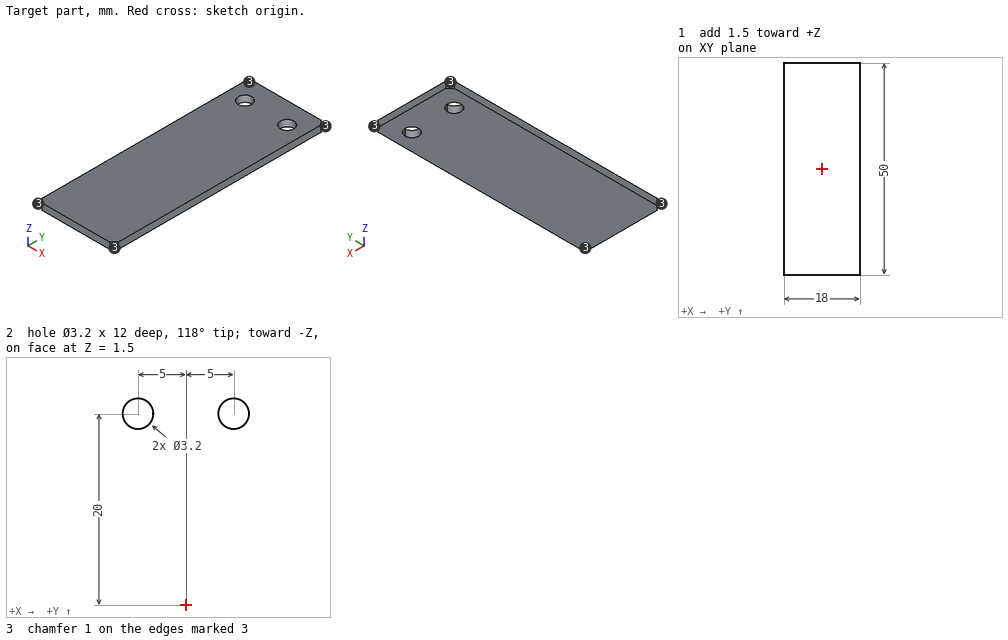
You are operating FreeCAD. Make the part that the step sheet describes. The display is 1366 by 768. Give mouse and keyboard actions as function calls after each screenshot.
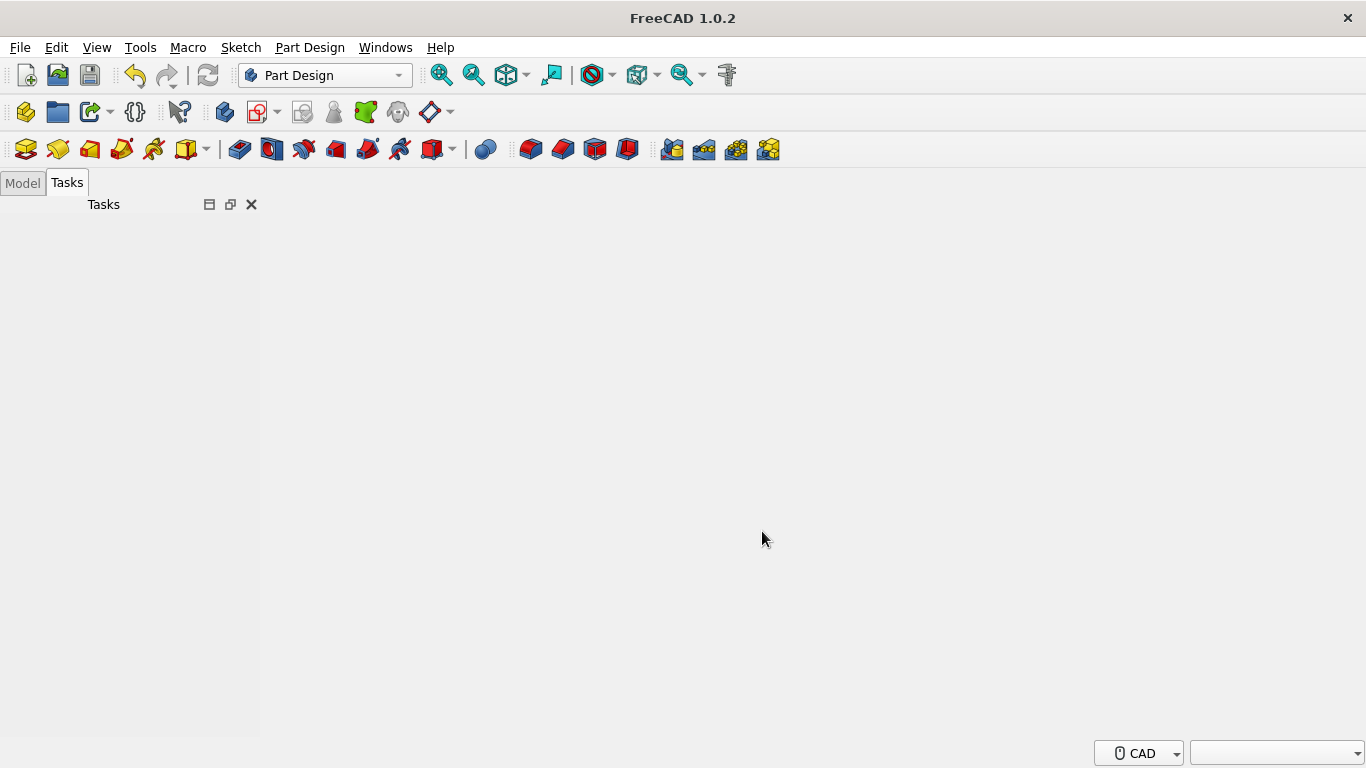
click(26, 76)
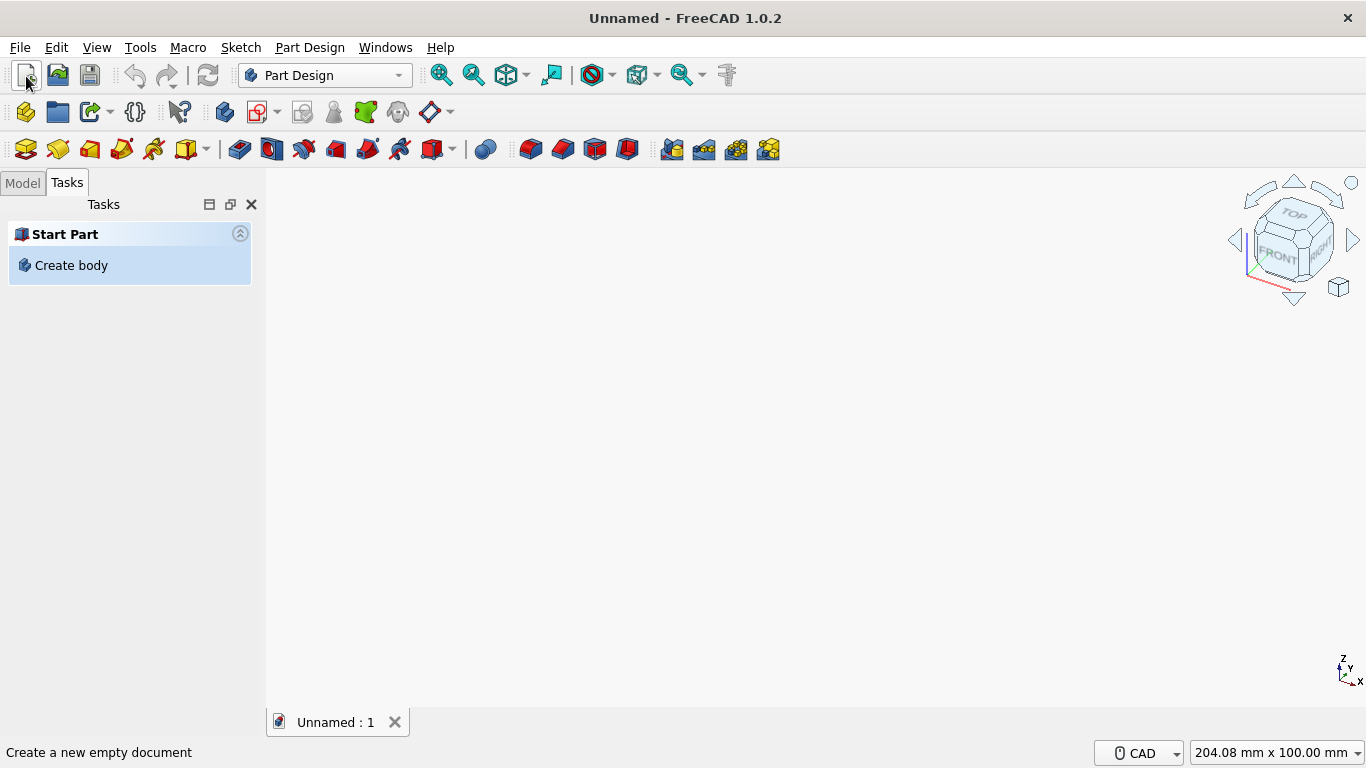
click(258, 112)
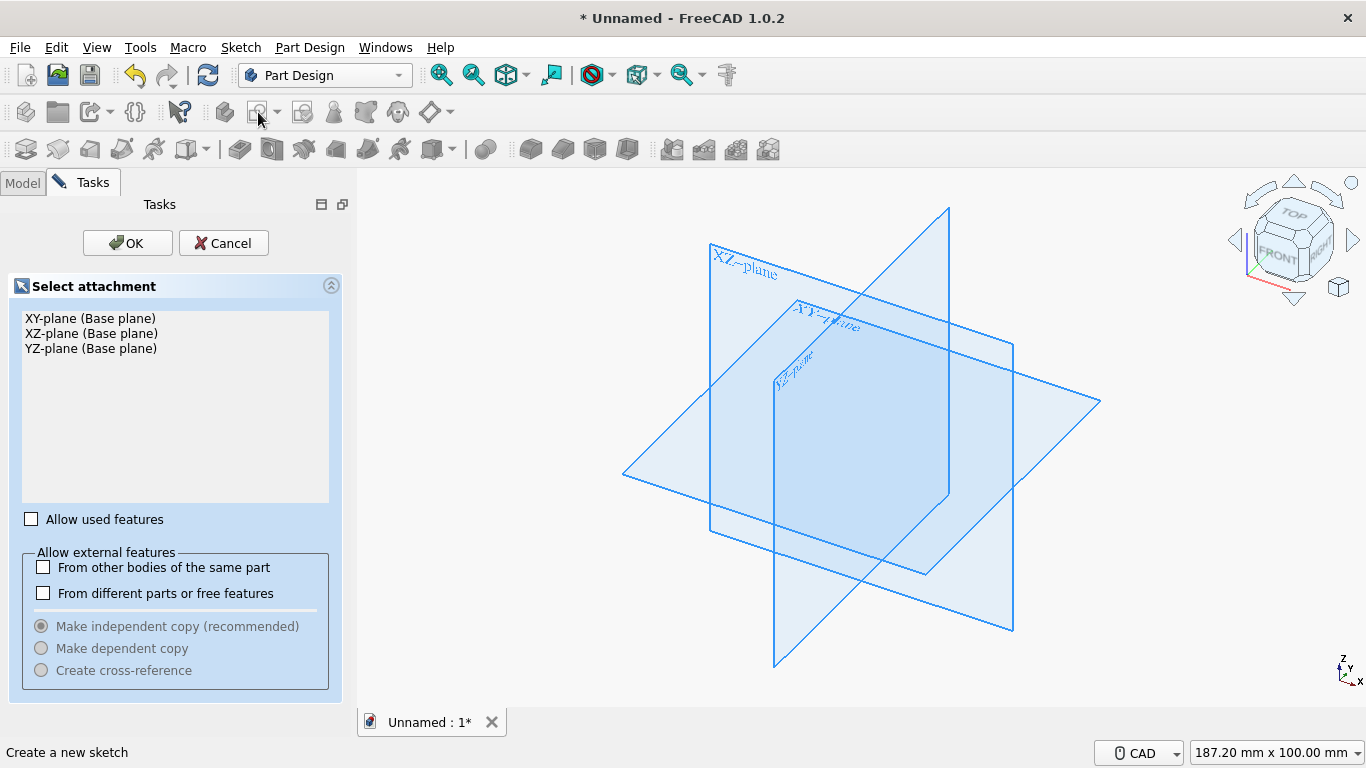
click(82, 318)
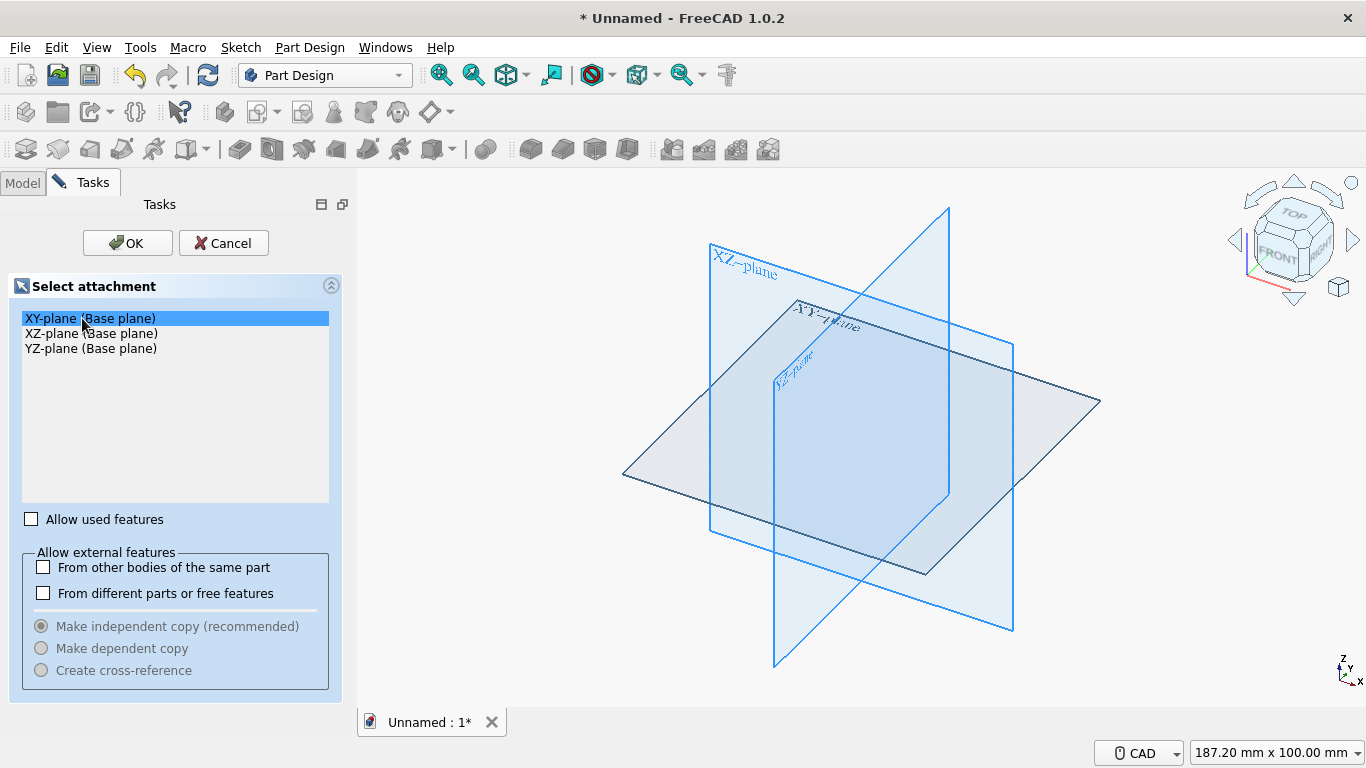
click(128, 243)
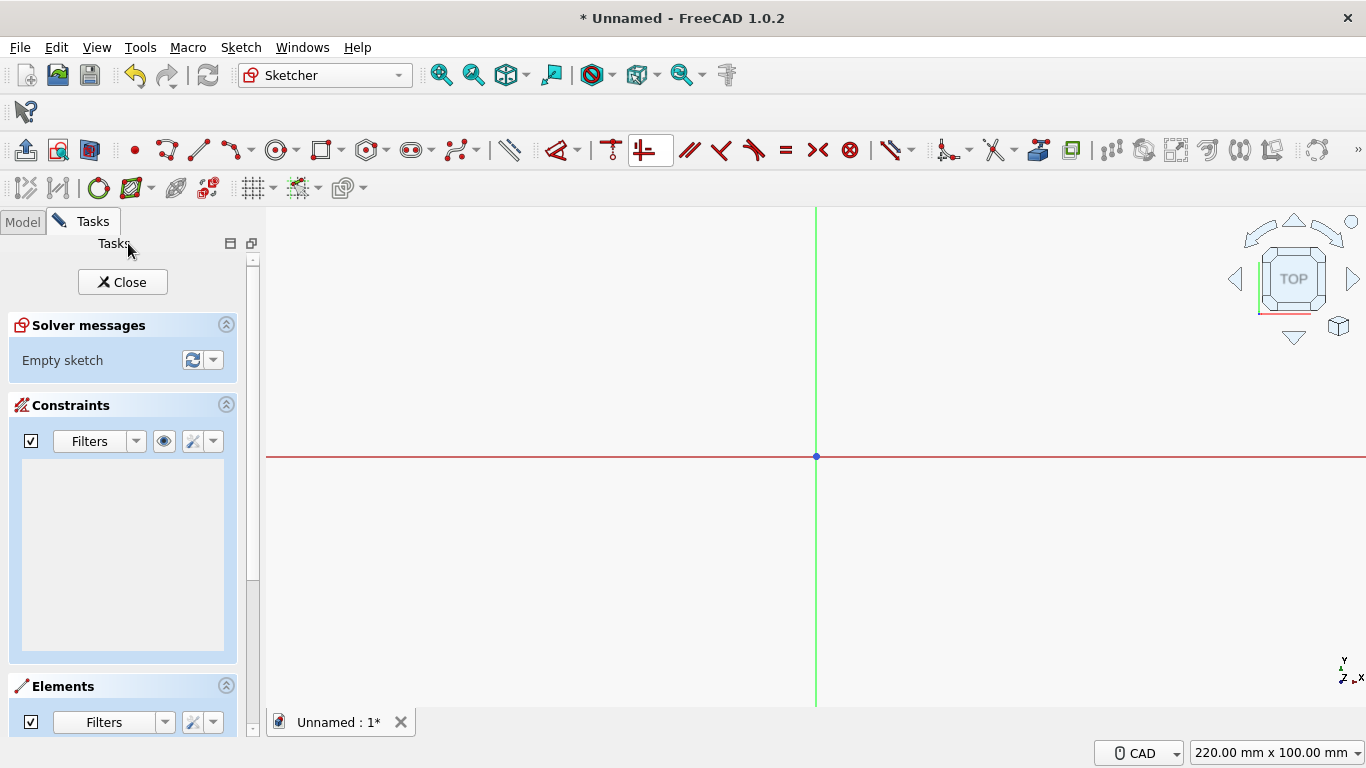
key(g)
key(v)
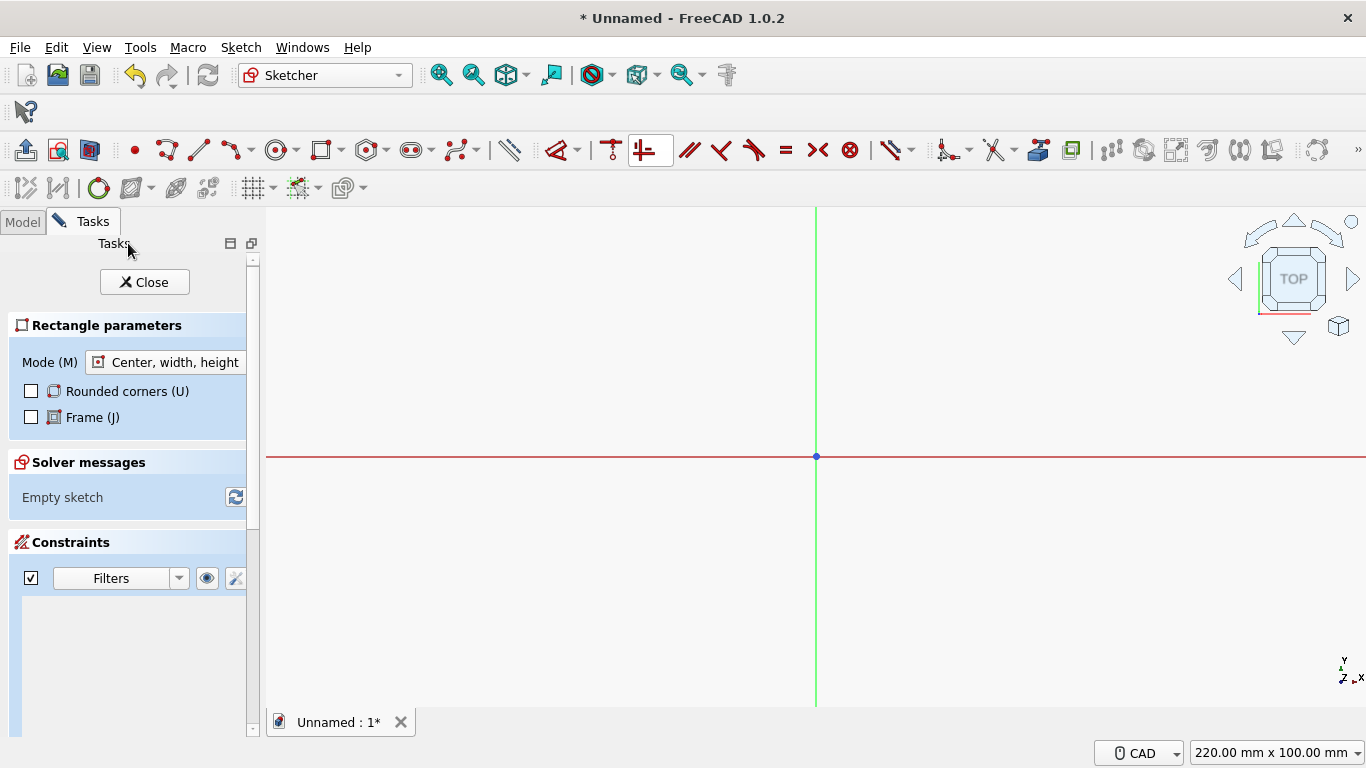
click(816, 457)
move(861, 332)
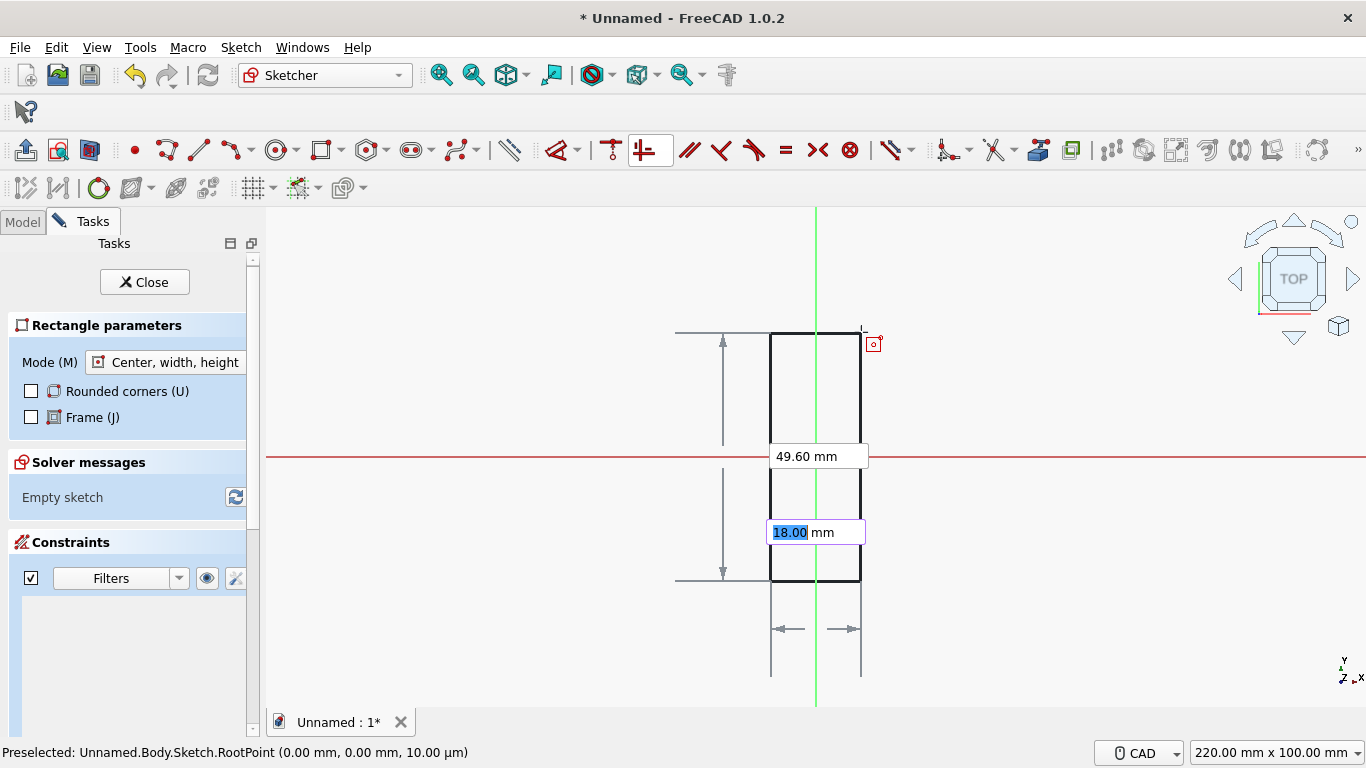
text(18)
key(Tab)
text(50)
key(Return)
key(Escape)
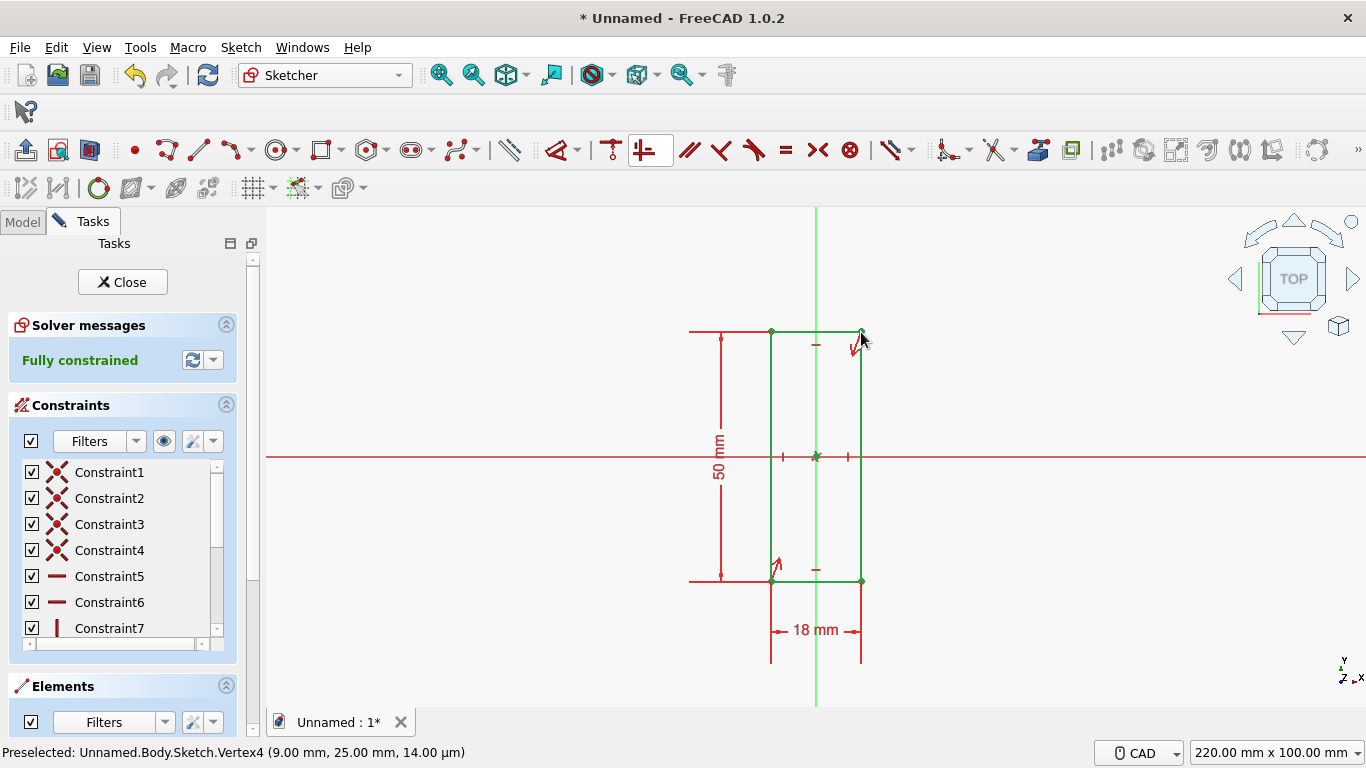
click(123, 282)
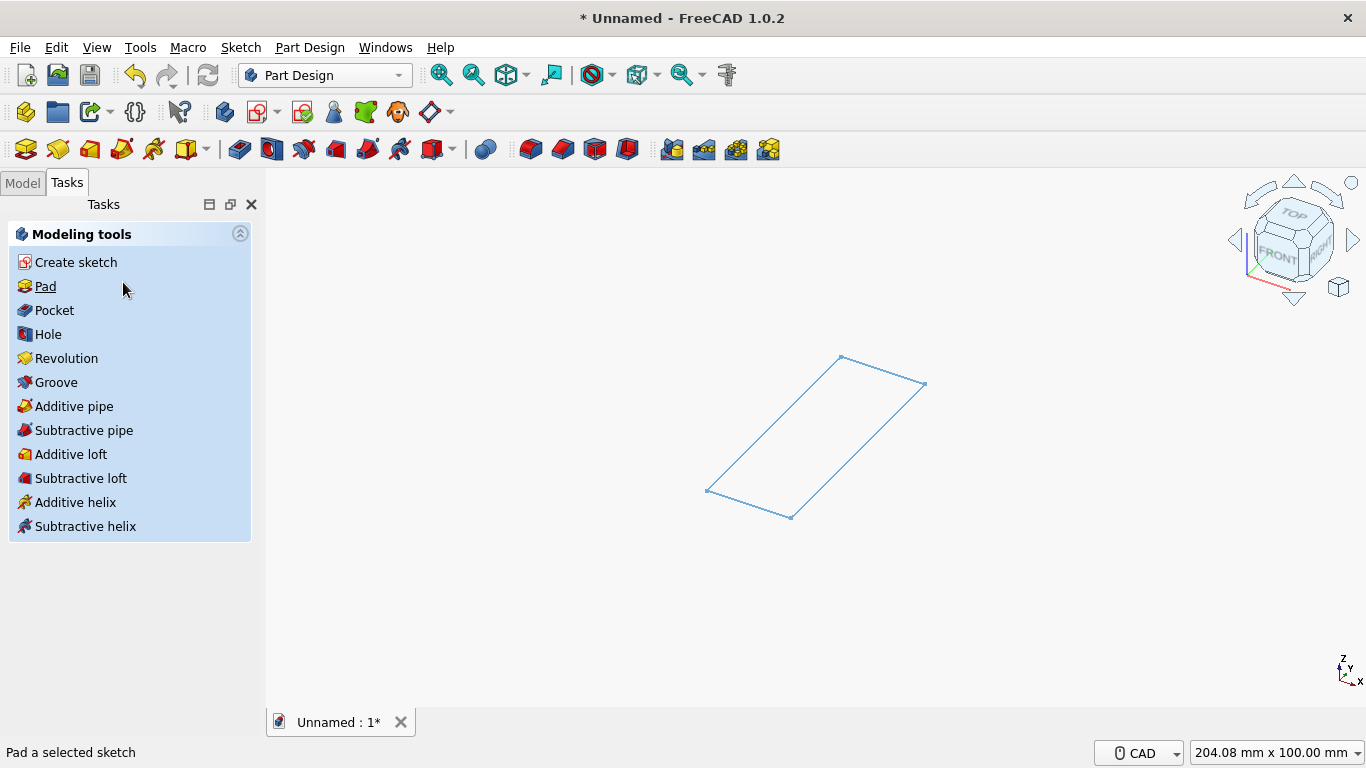
click(26, 150)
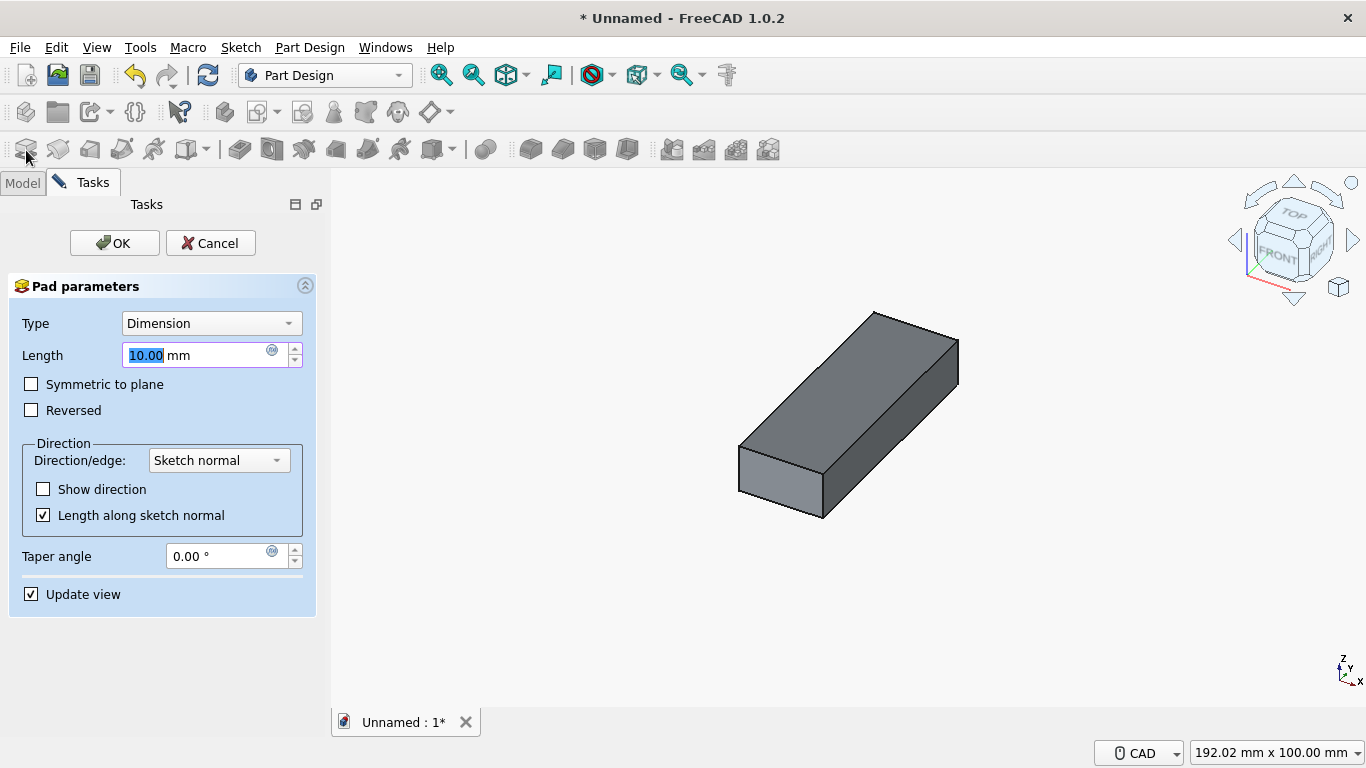
text(1.5)
key(Tab)